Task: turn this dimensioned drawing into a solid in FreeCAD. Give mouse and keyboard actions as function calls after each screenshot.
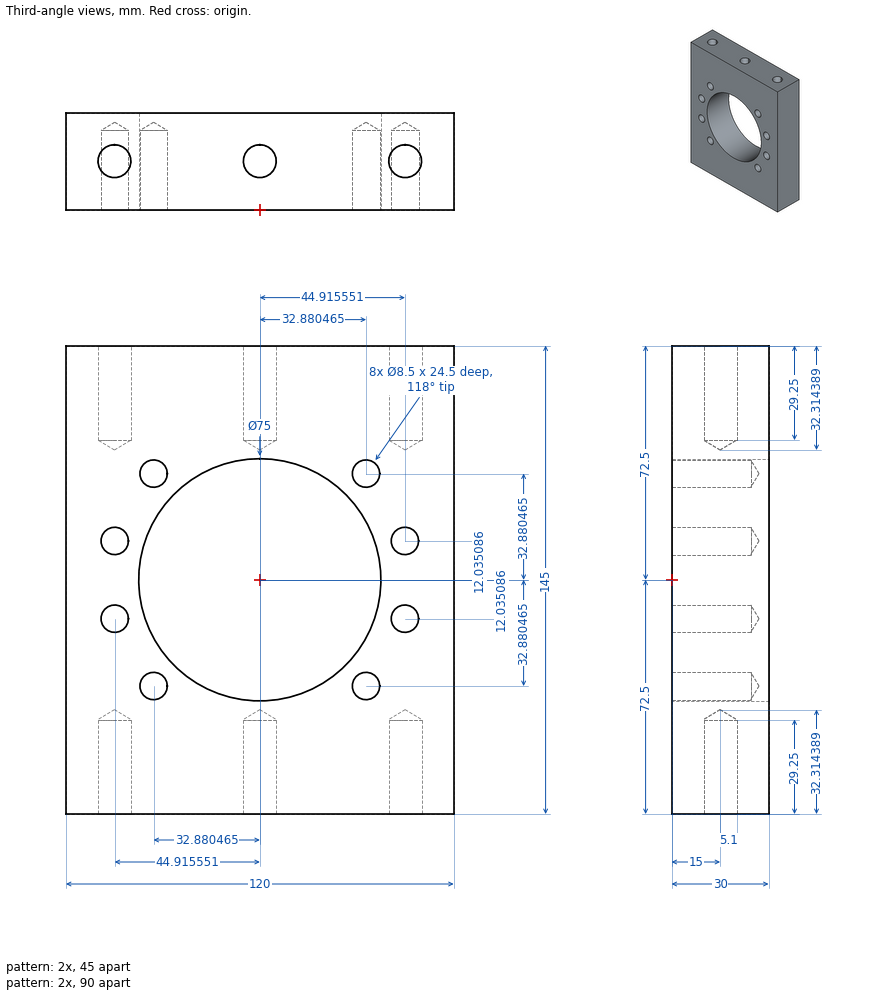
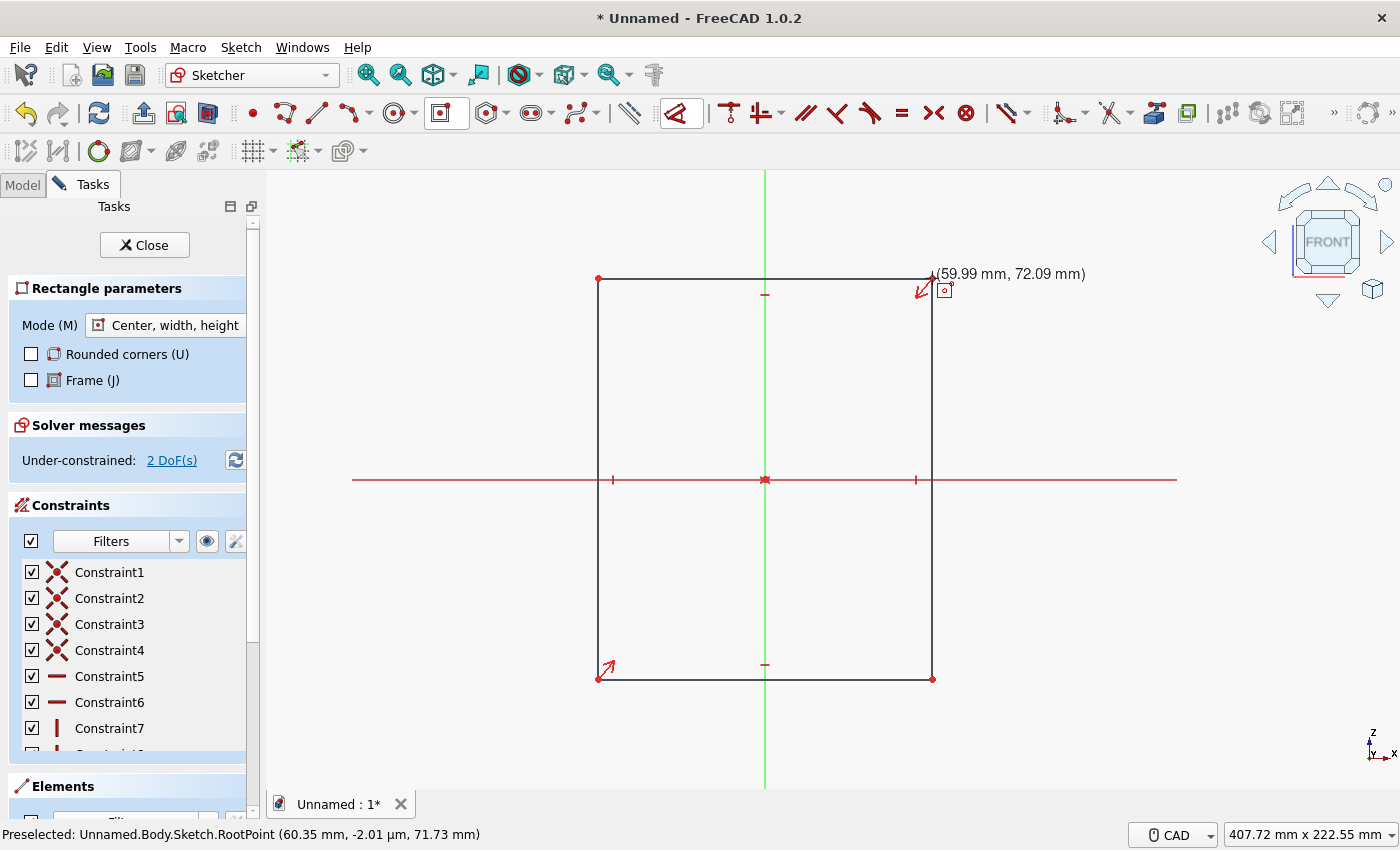
click(394, 114)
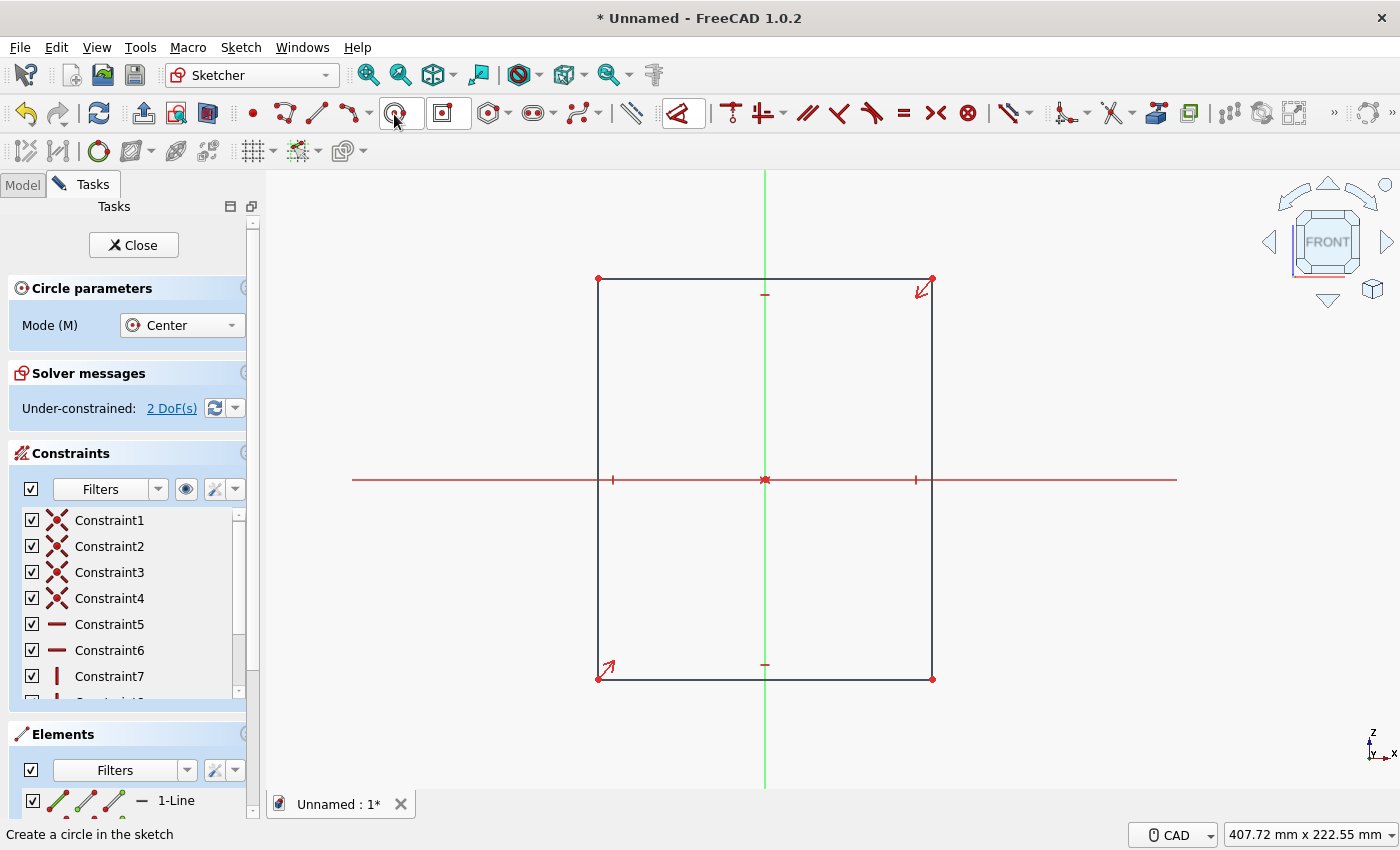
click(765, 480)
click(839, 406)
key(Escape)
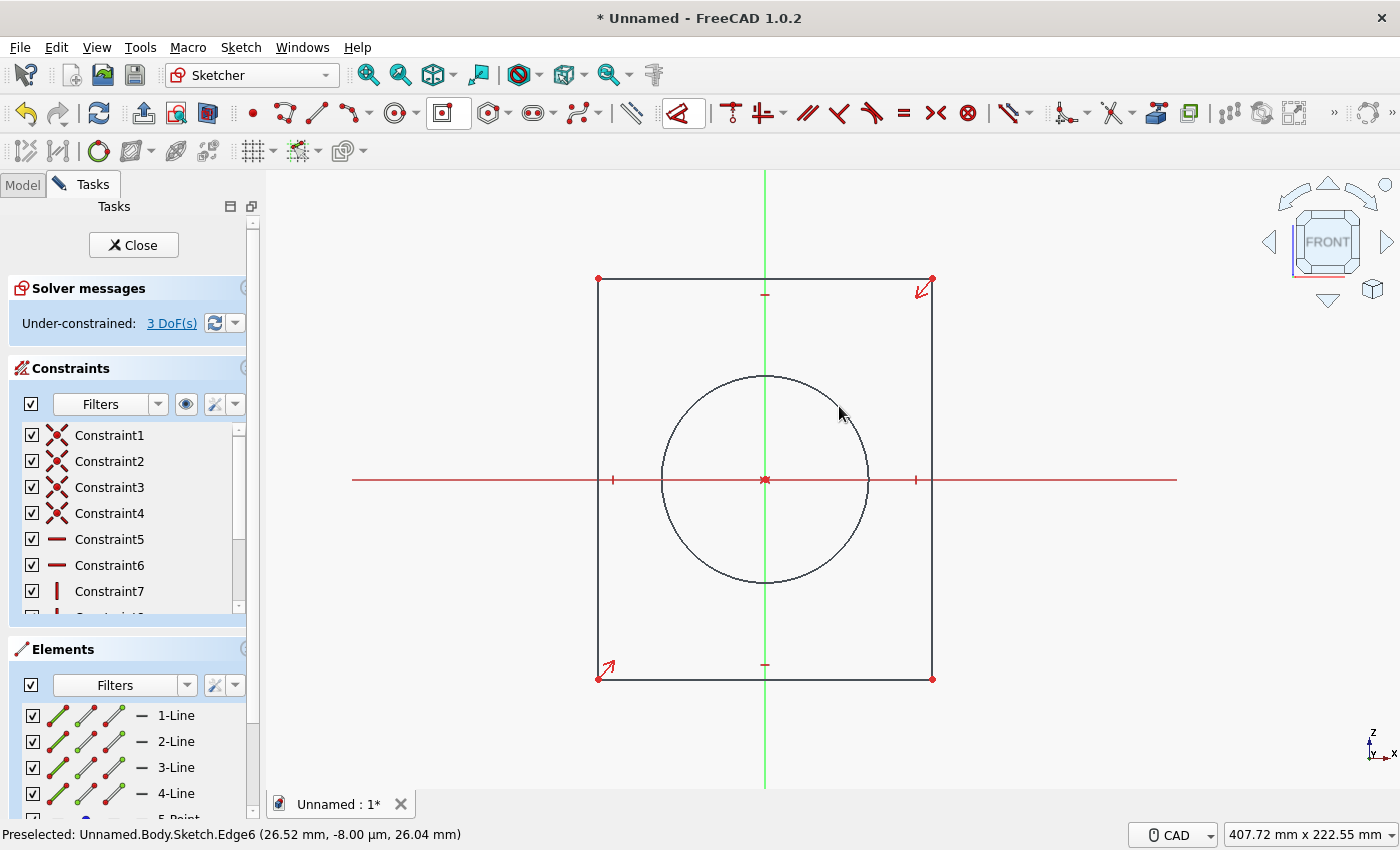
click(678, 114)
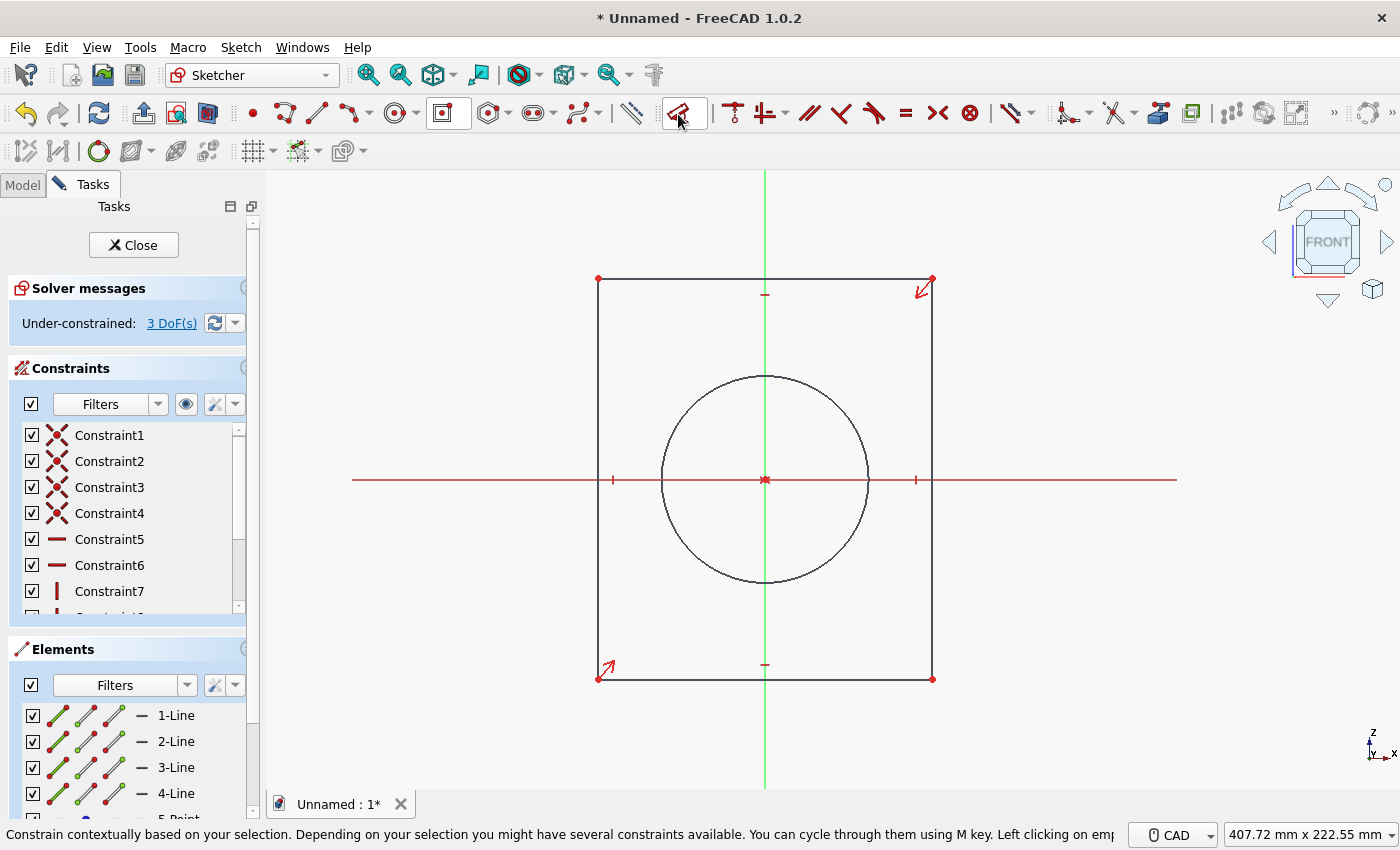
click(838, 406)
click(861, 383)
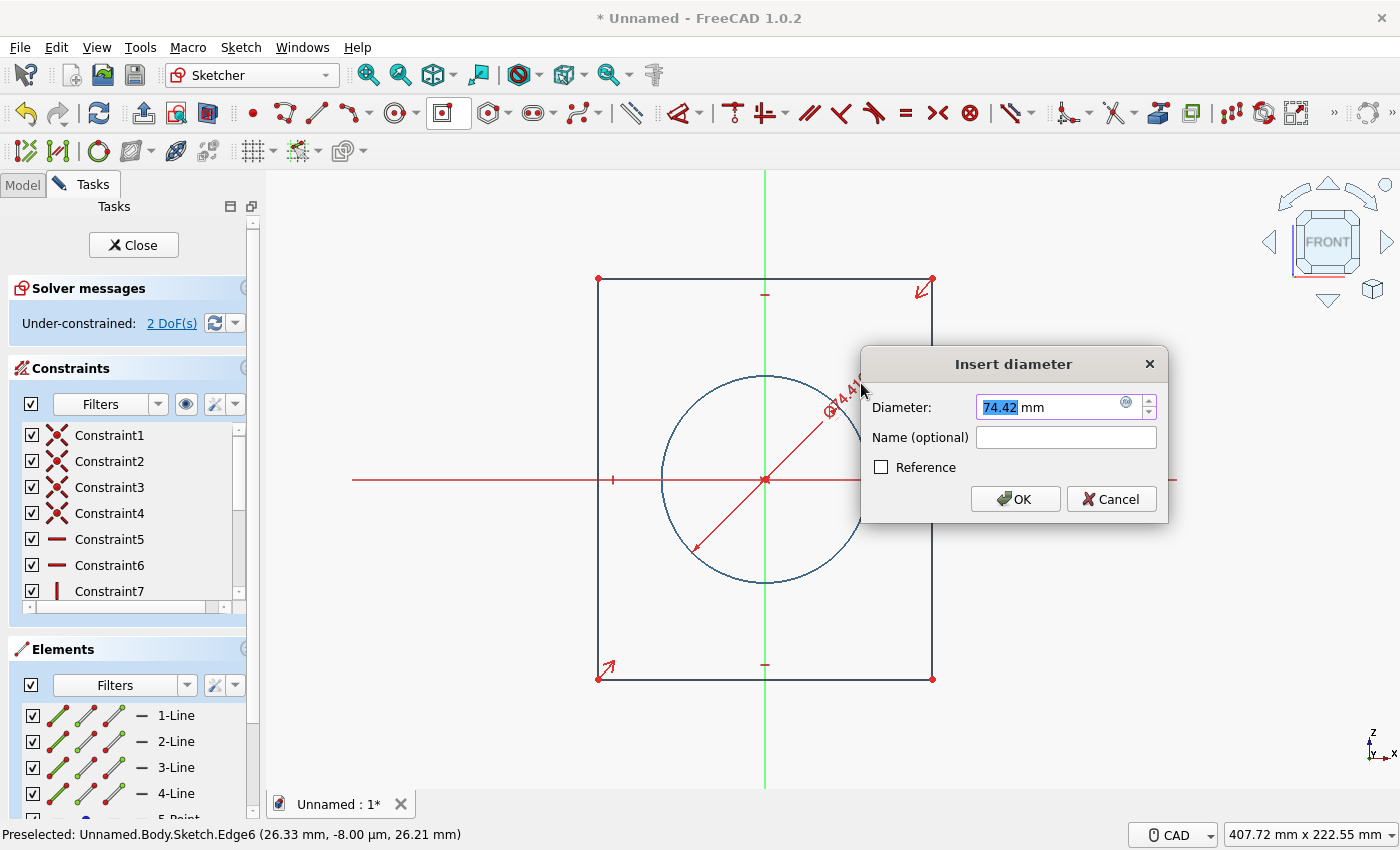
text(75)
key(Return)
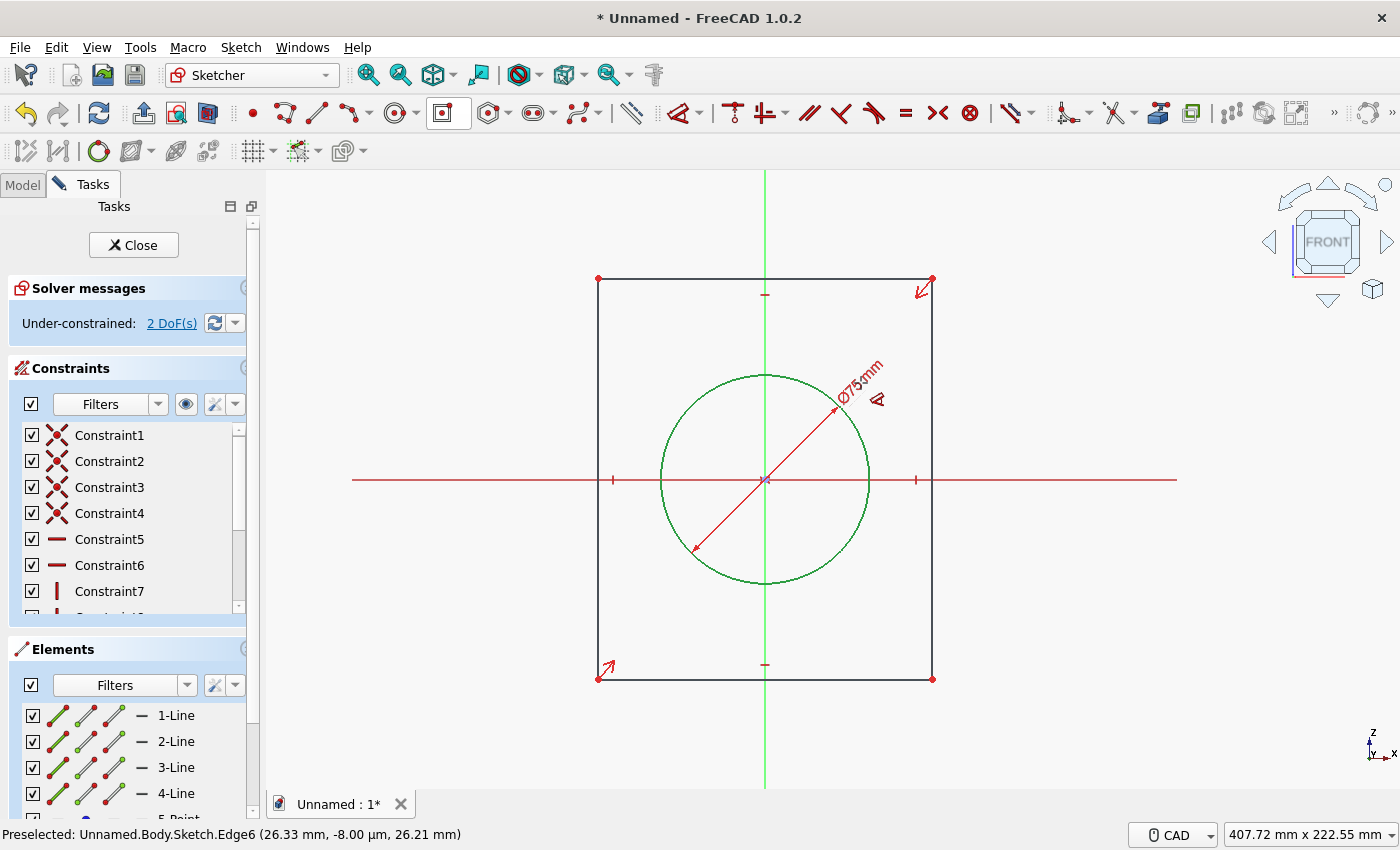
click(698, 680)
click(688, 714)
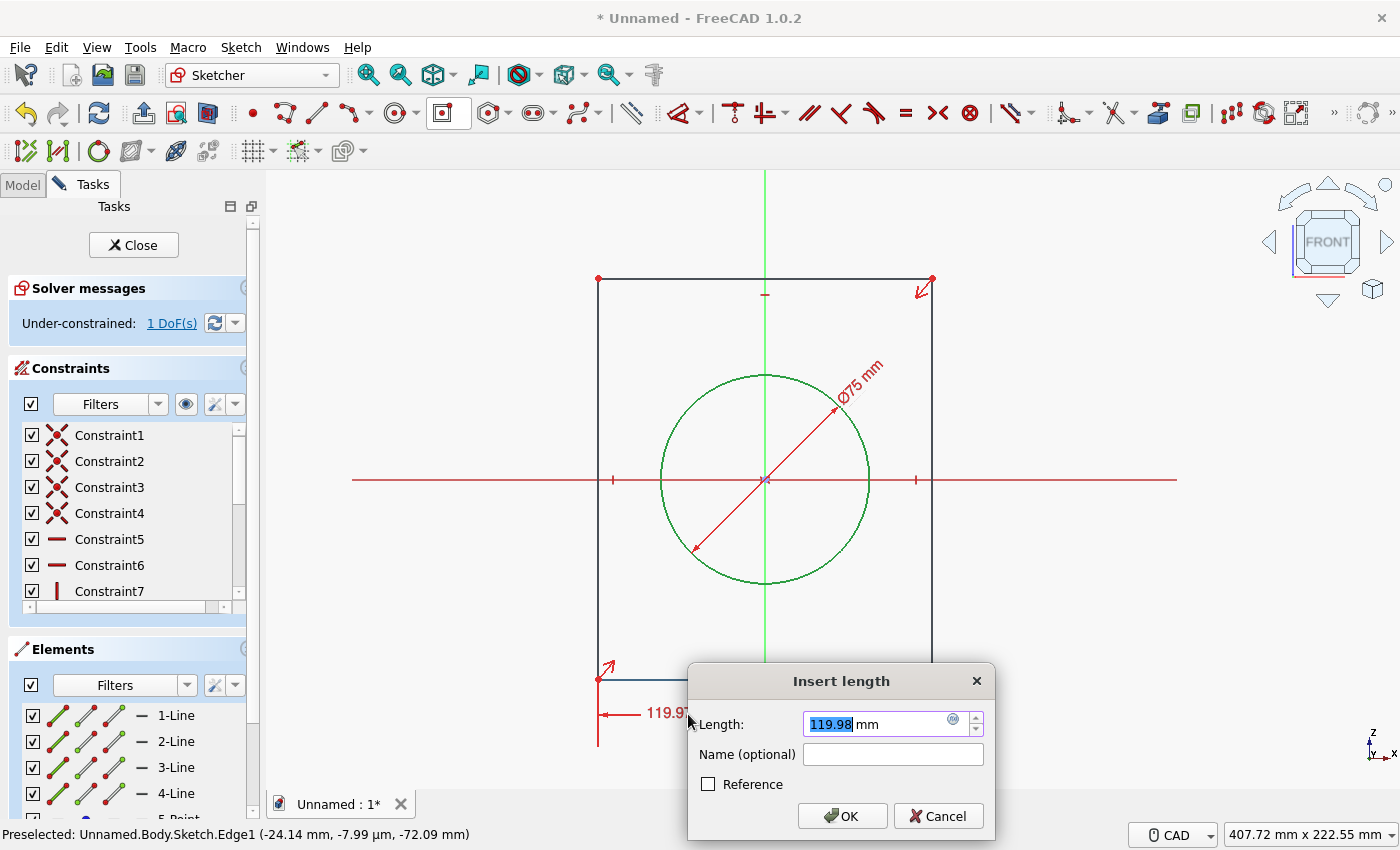
text(120)
key(Return)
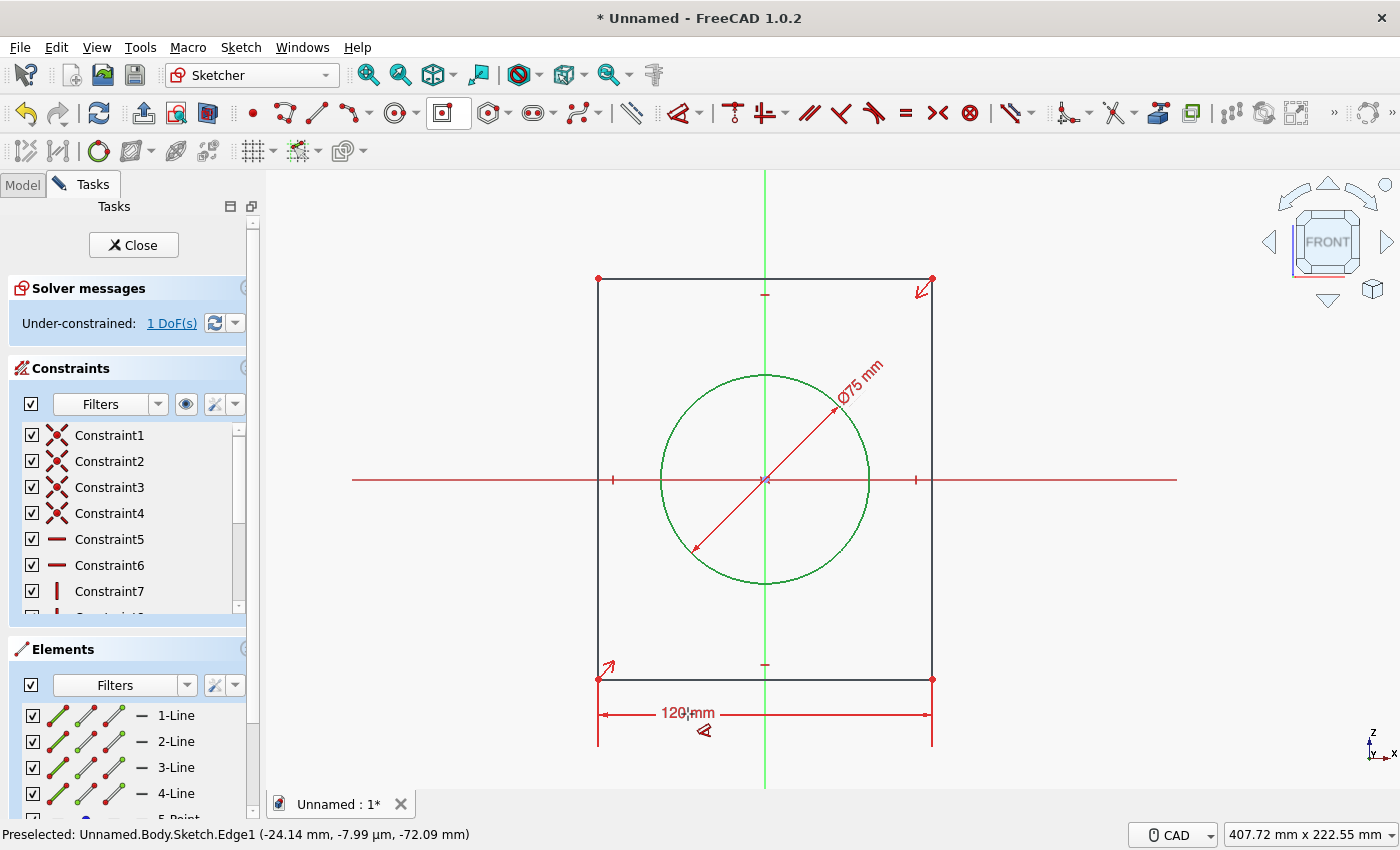
click(932, 560)
click(966, 387)